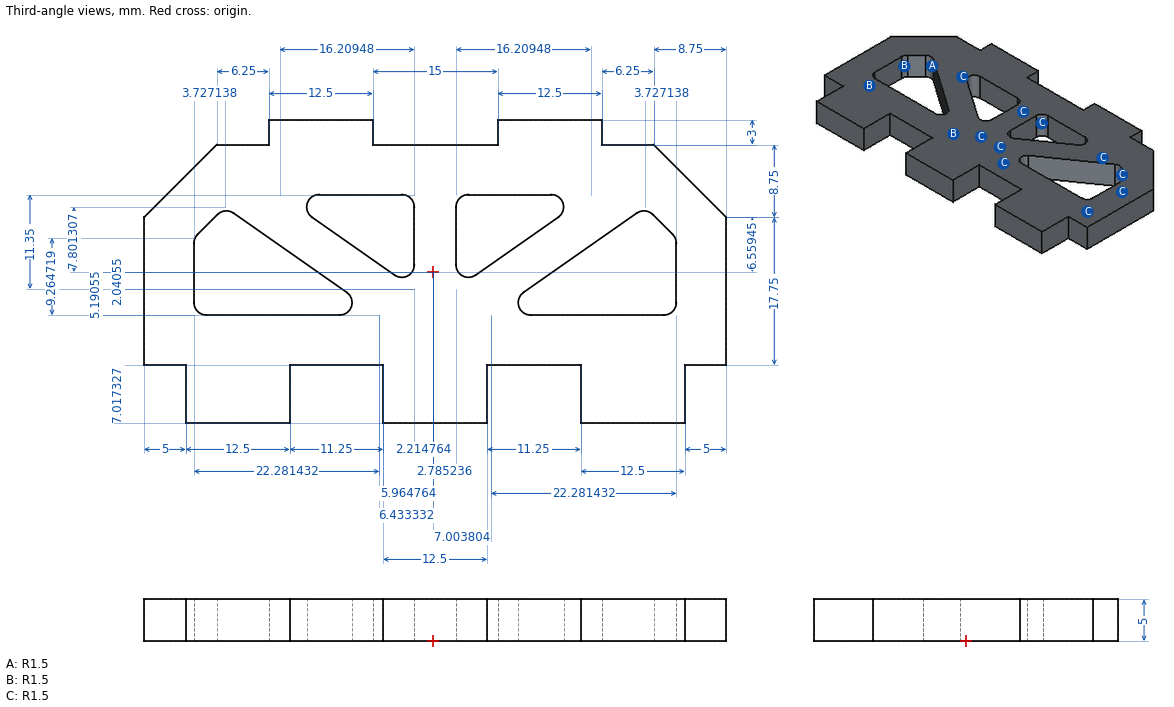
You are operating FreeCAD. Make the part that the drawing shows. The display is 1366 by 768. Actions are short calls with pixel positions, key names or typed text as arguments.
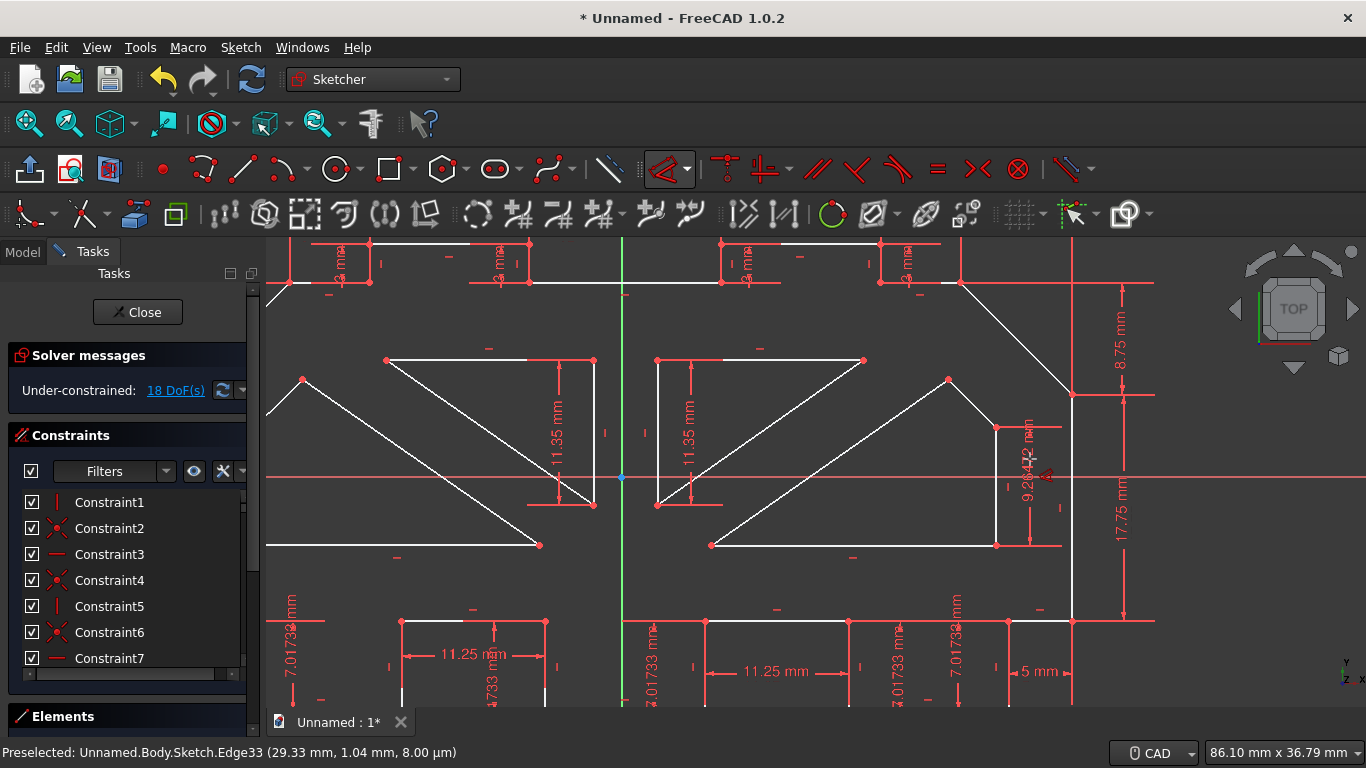
click(448, 360)
click(490, 326)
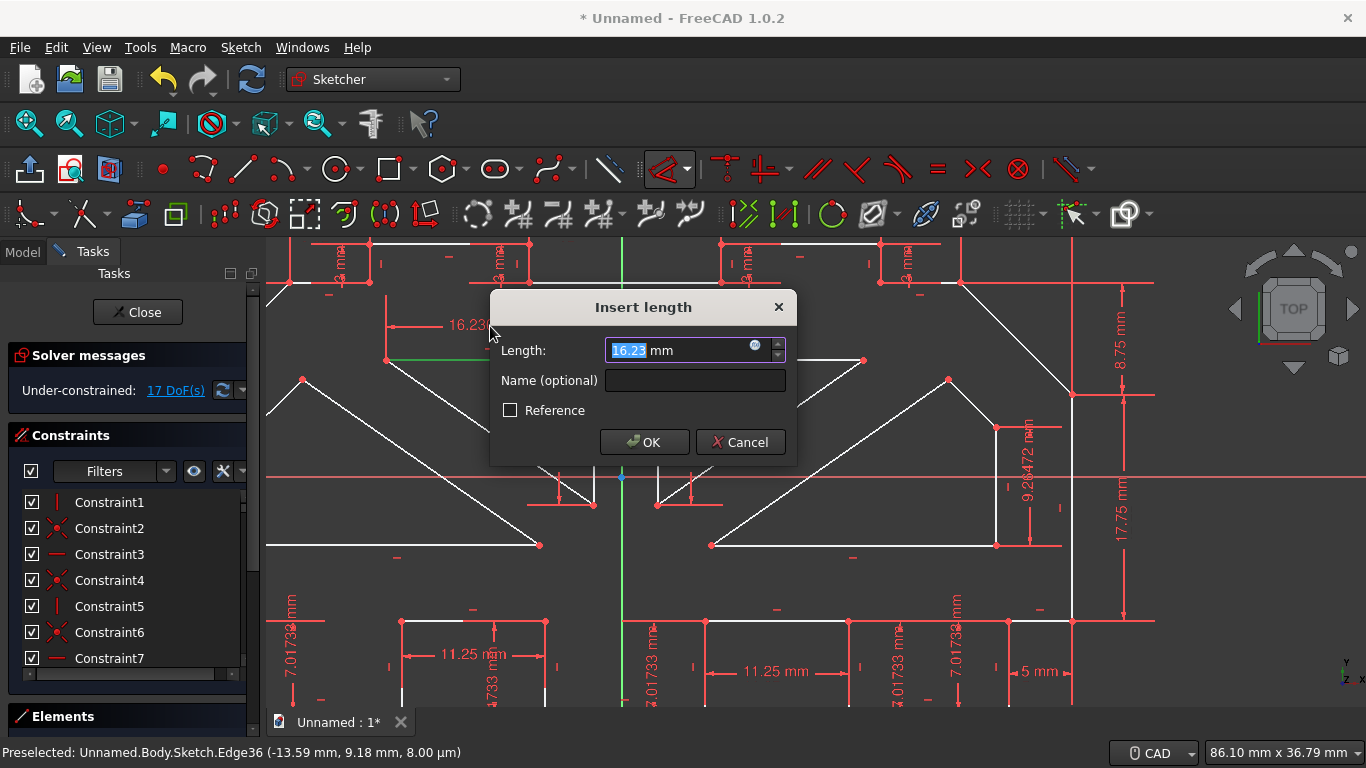
text(16.20948)
key(Return)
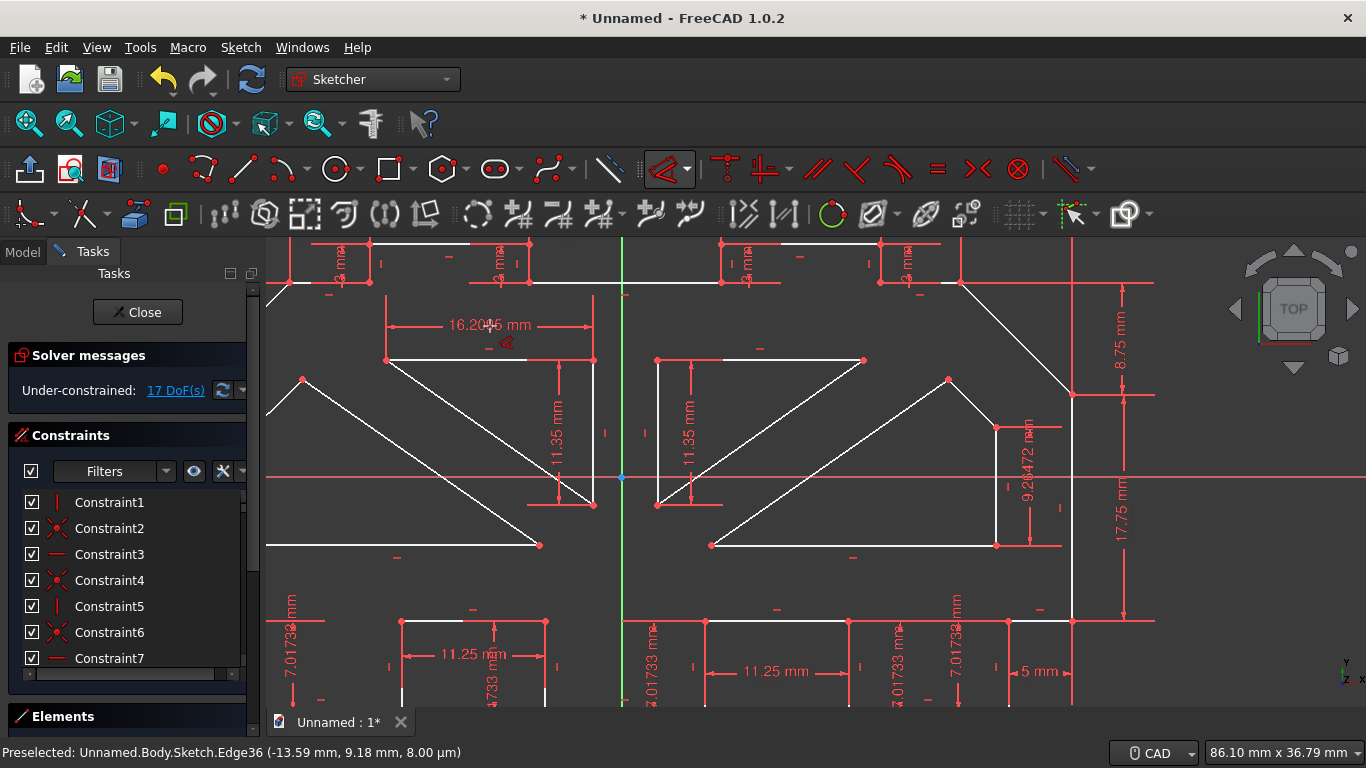
click(719, 360)
click(761, 326)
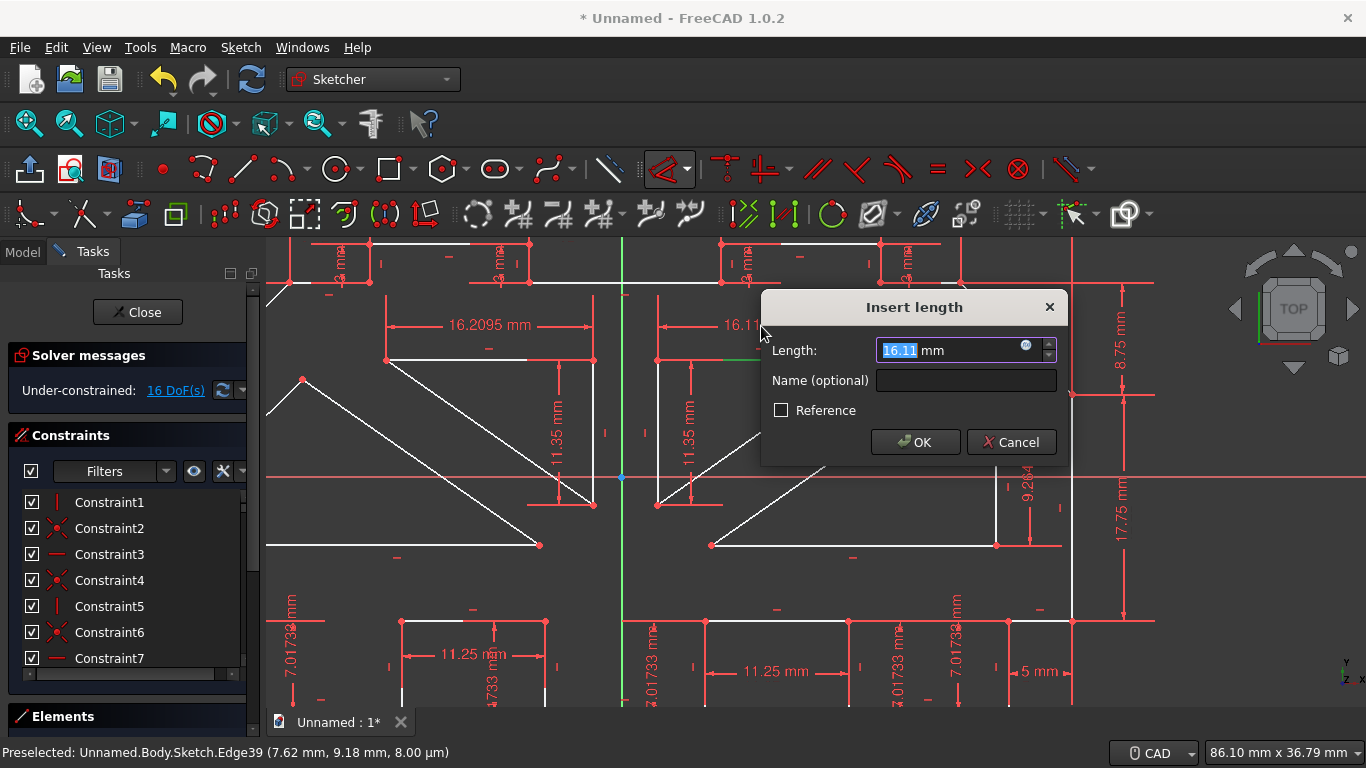
text(16.20948)
key(Return)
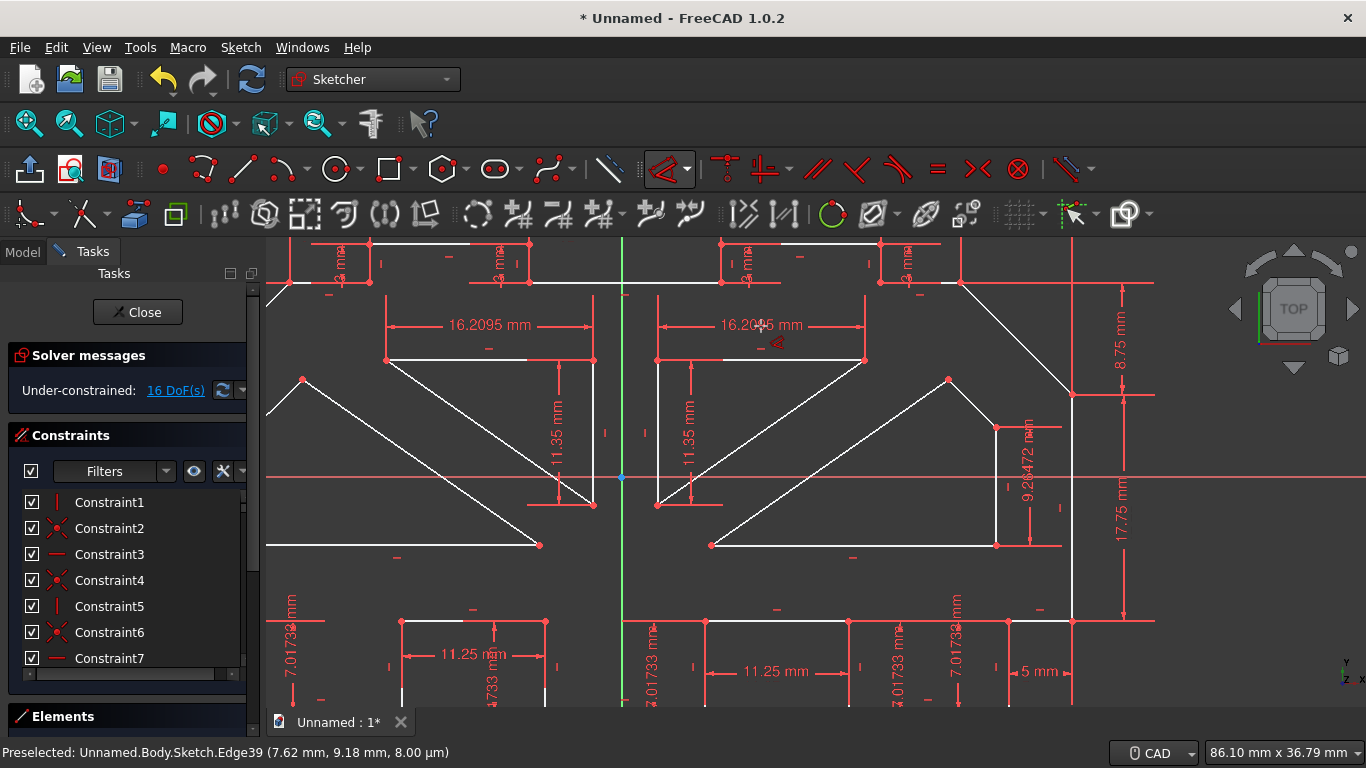
click(1072, 395)
click(1106, 436)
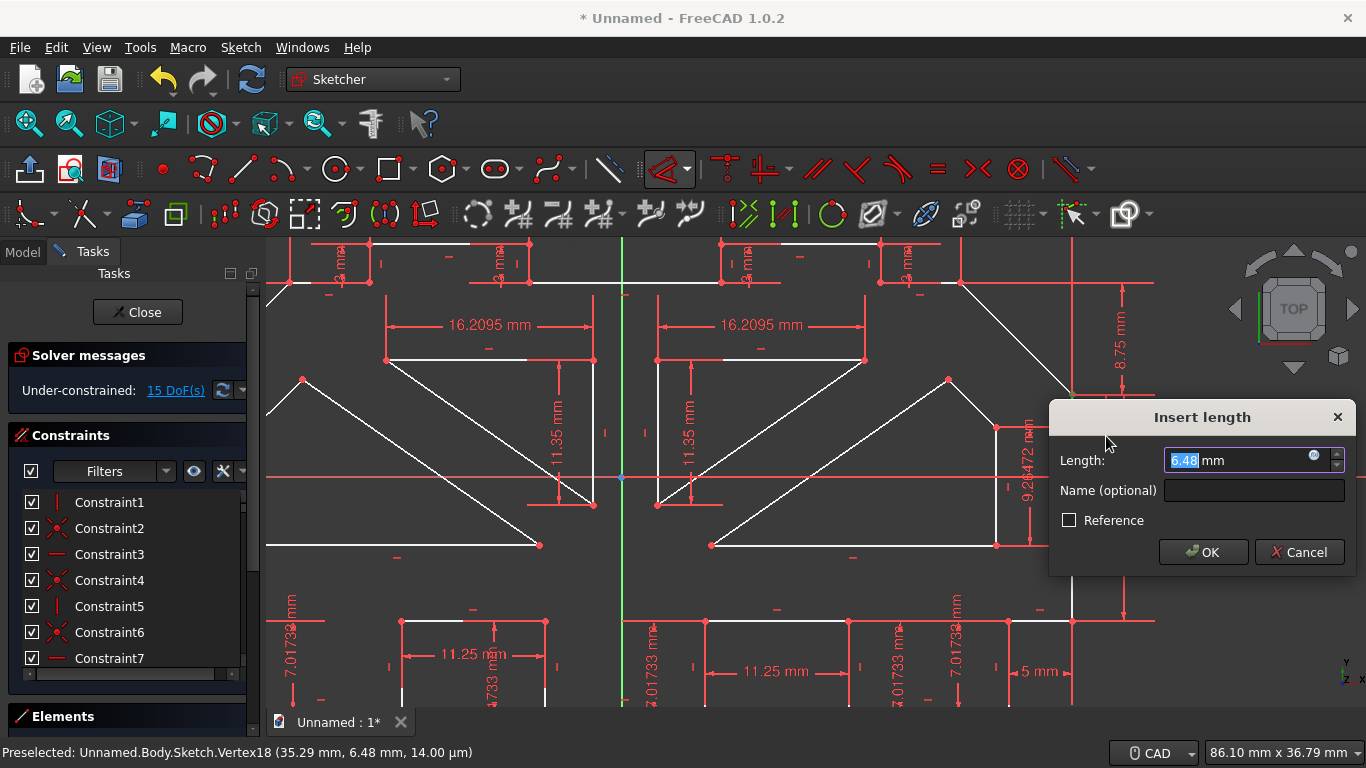
text(6.55945)
key(Return)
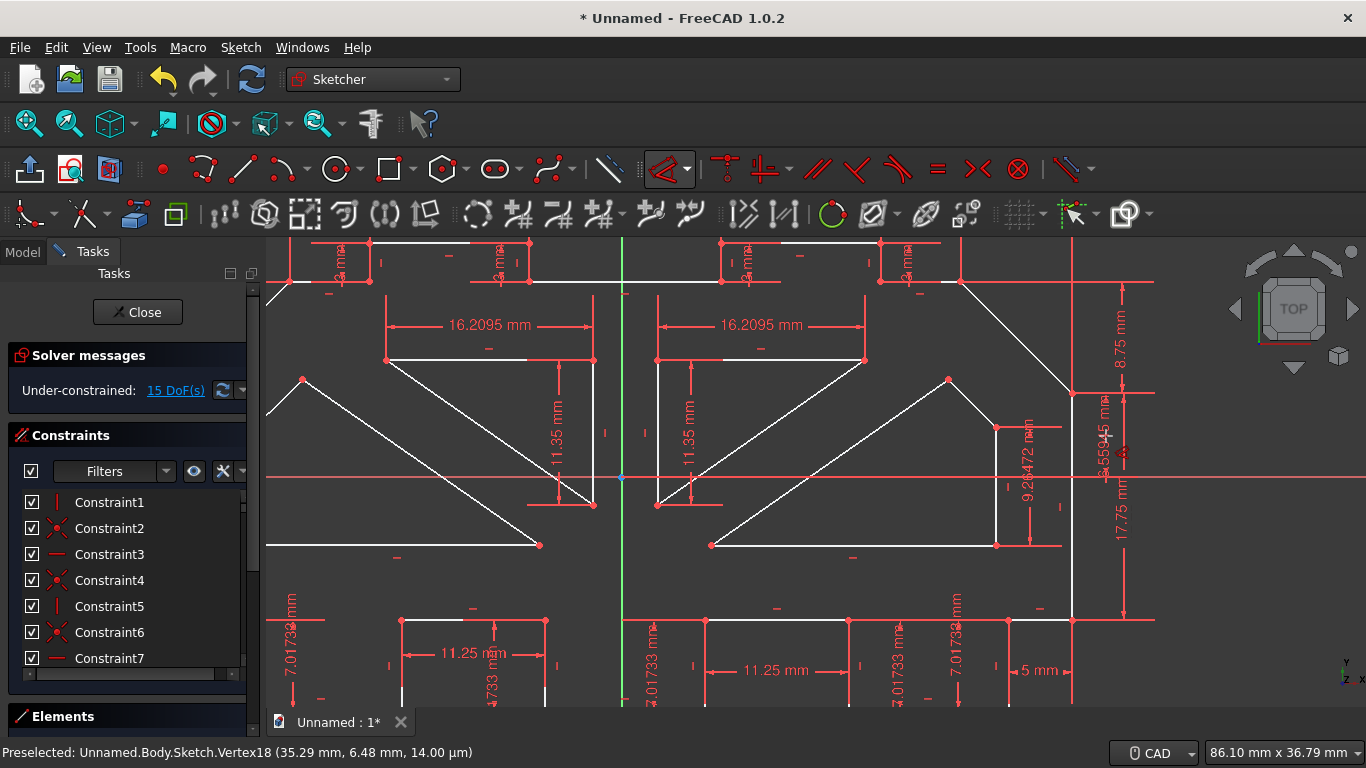
click(540, 545)
click(506, 496)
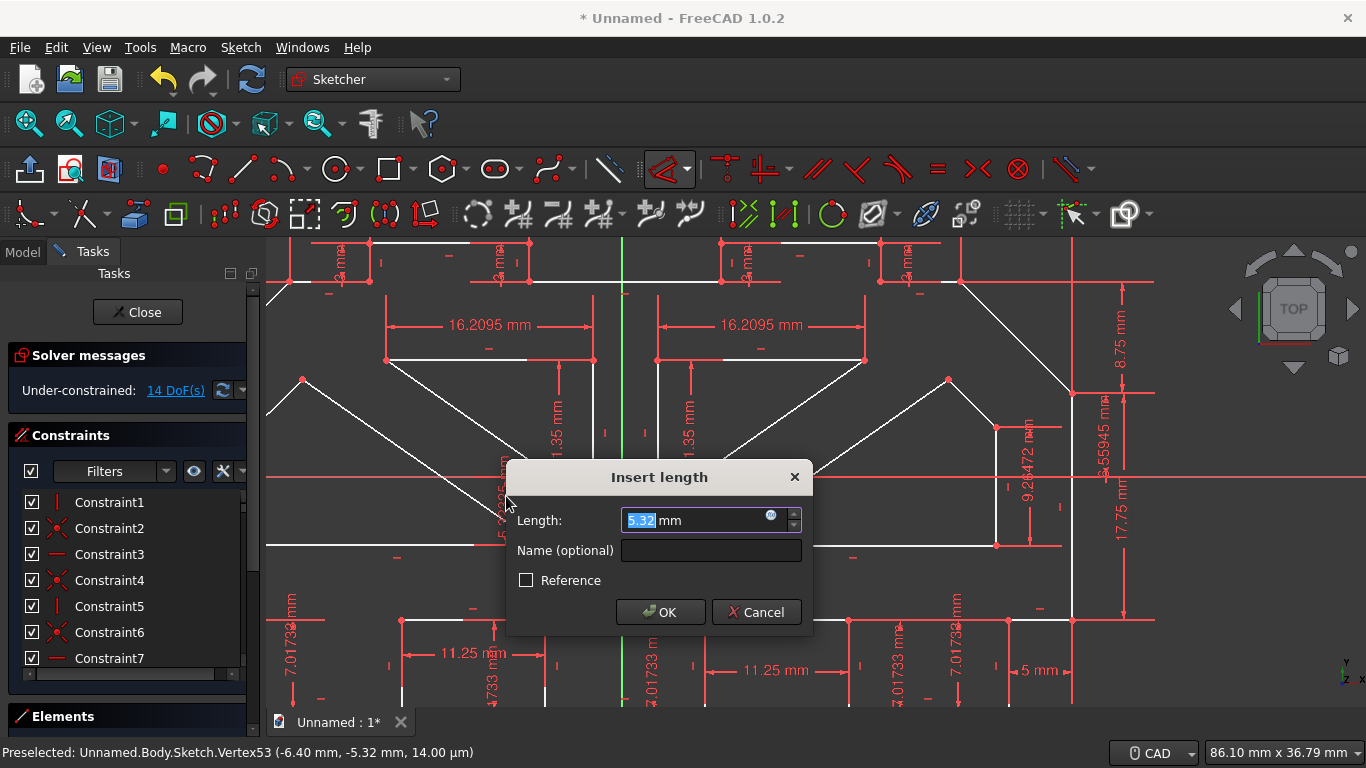
text(5.19055)
key(Return)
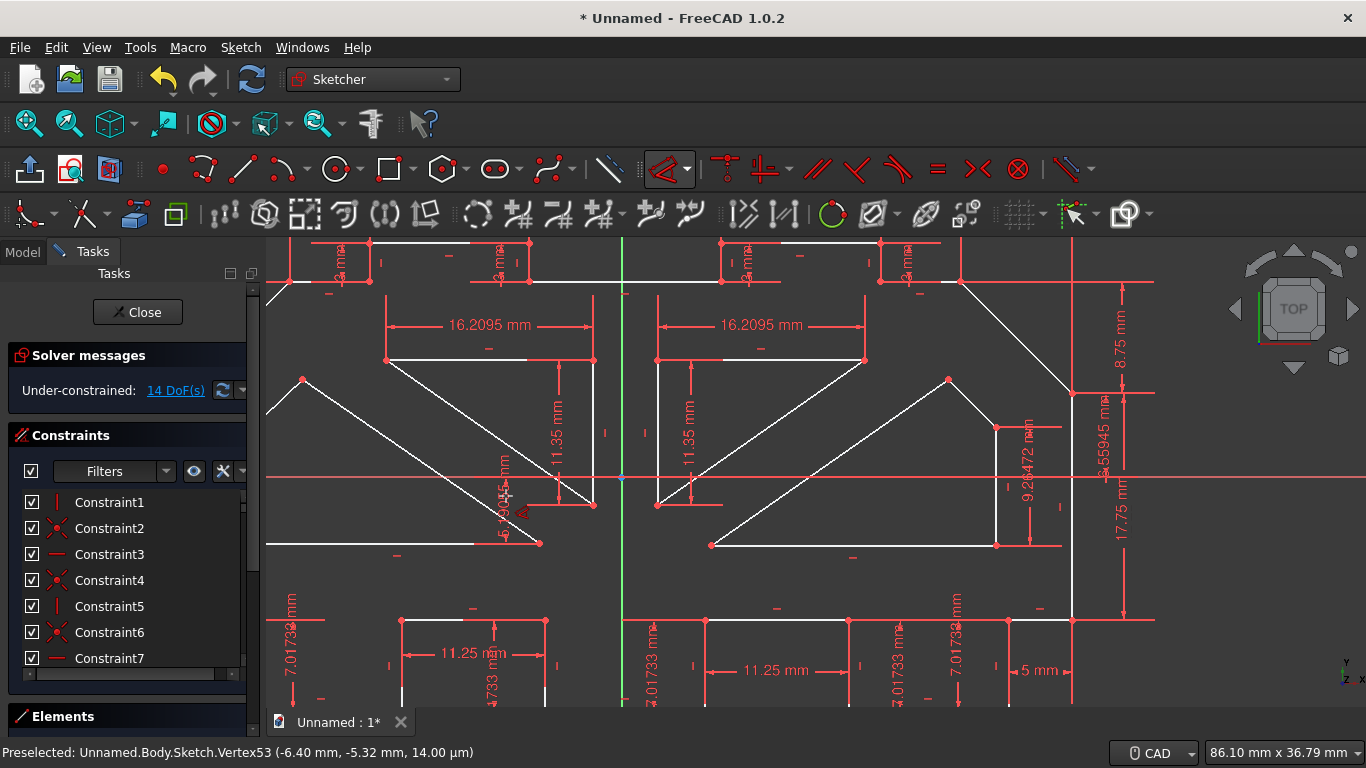
click(711, 546)
click(745, 496)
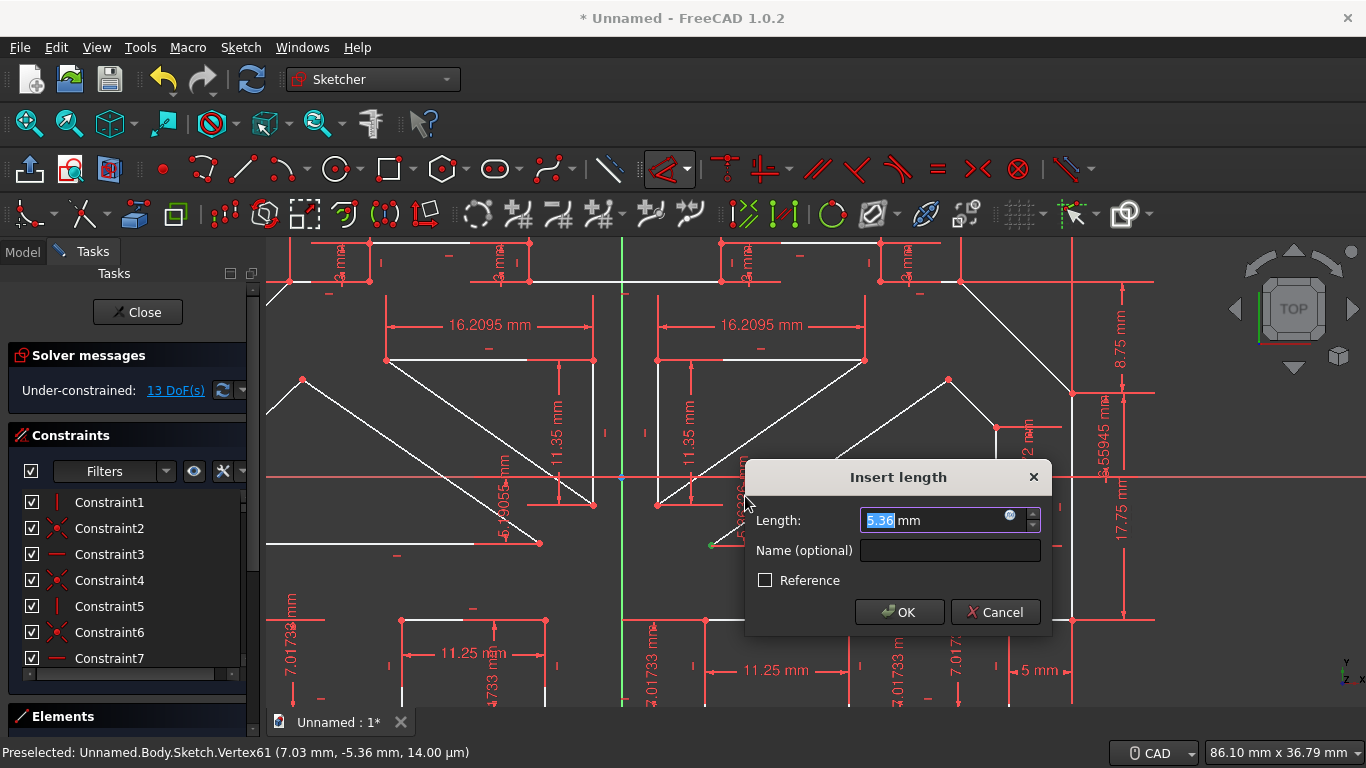
text(5.19055)
key(Return)